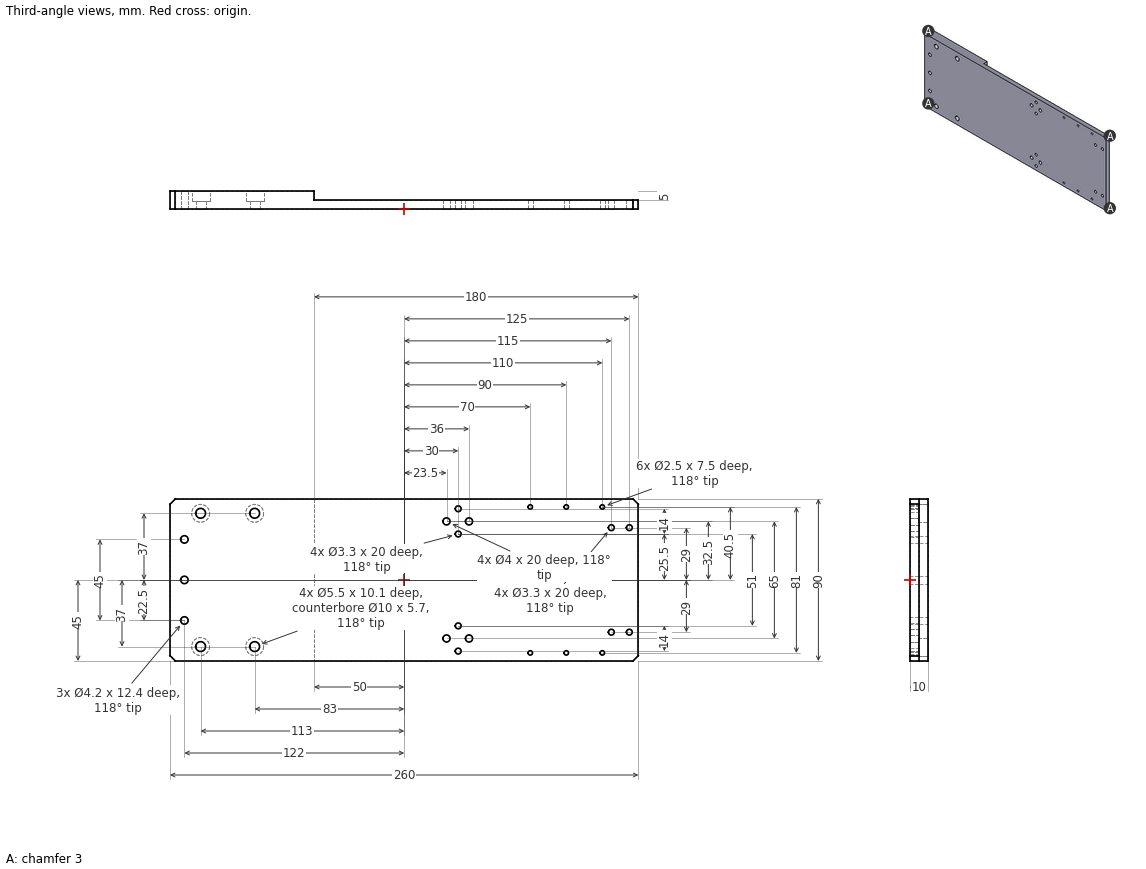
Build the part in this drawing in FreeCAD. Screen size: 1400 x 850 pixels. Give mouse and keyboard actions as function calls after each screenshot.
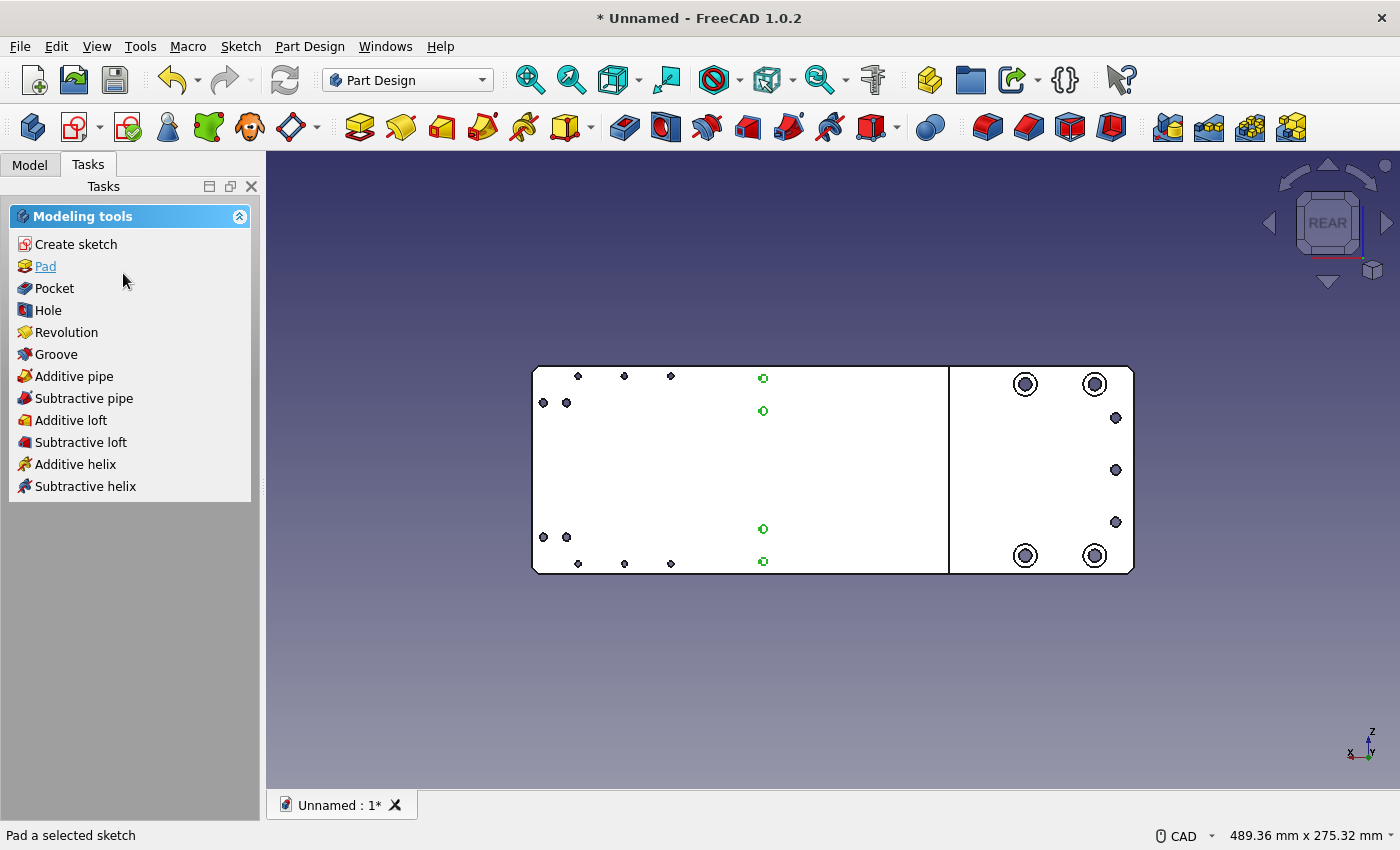
click(666, 128)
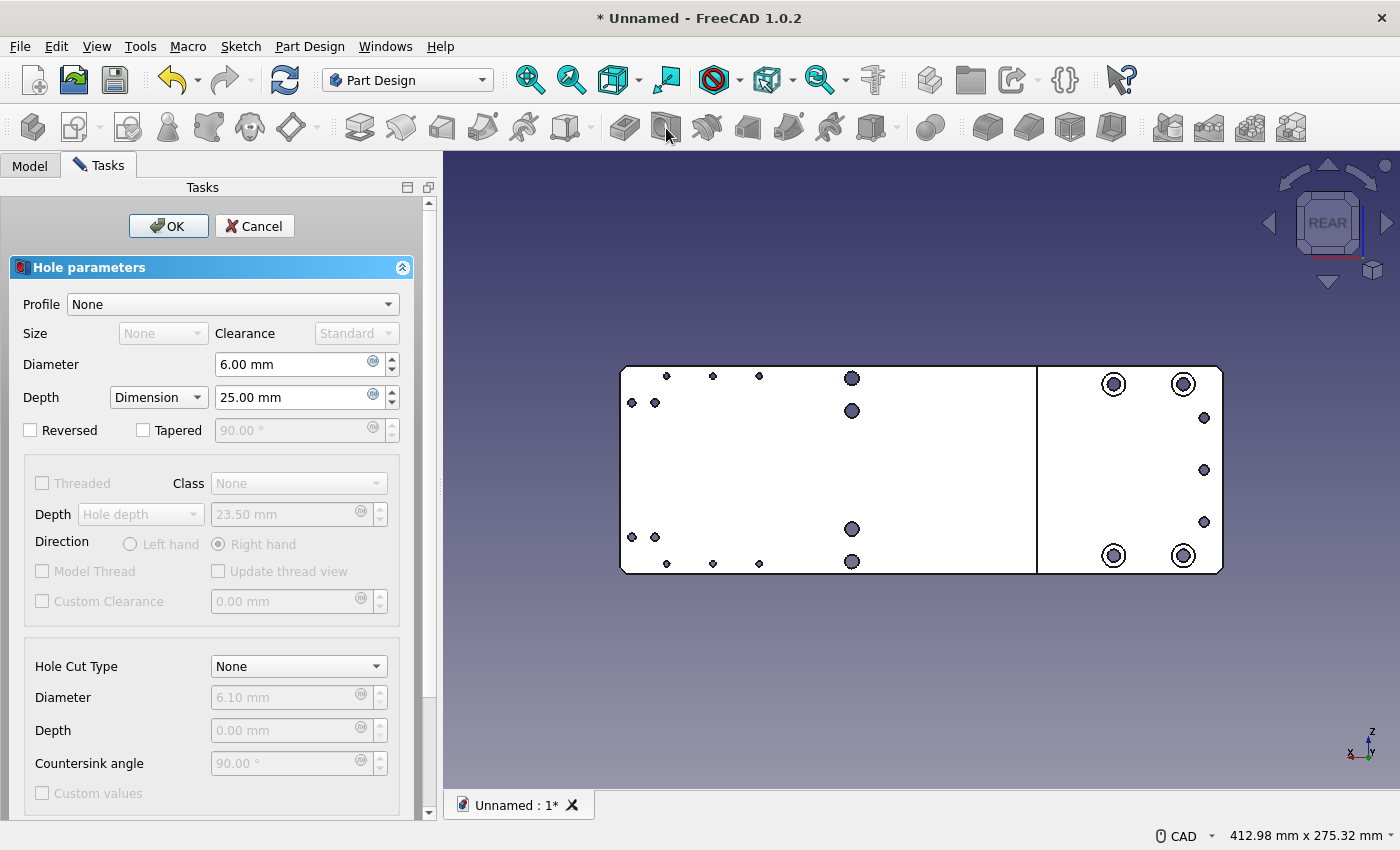
triple_click(300, 364)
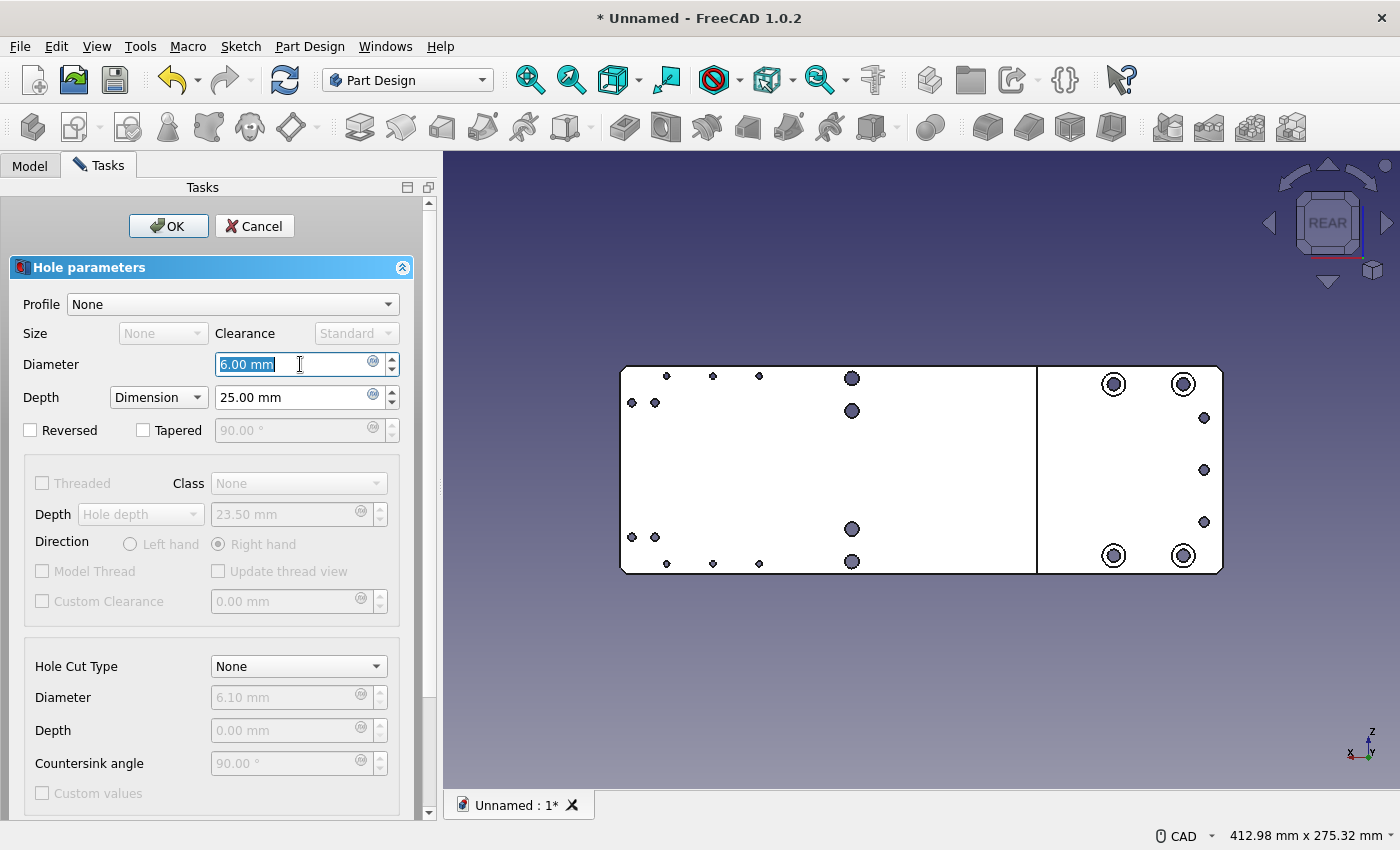
text(3.3)
key(Tab)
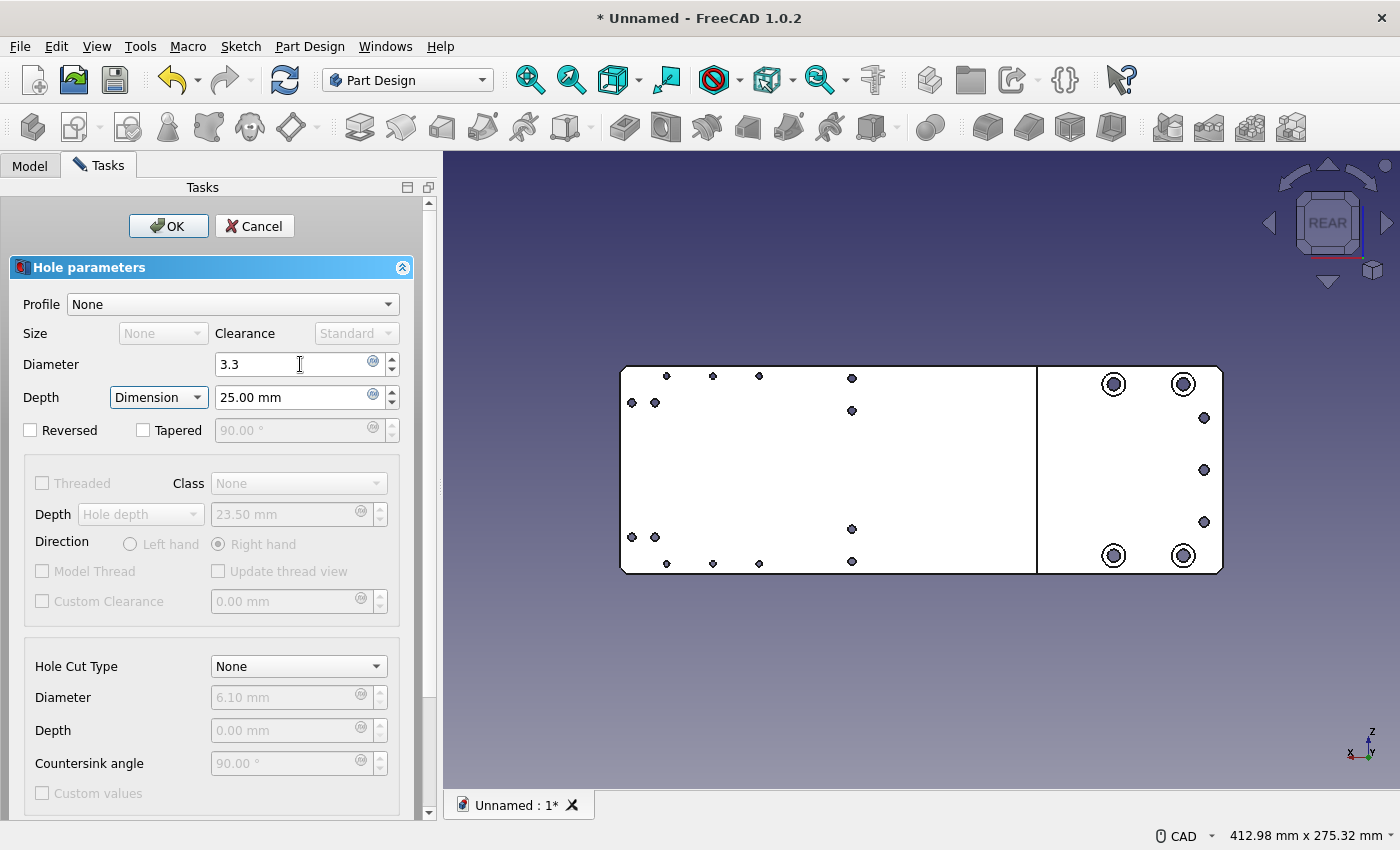
triple_click(300, 398)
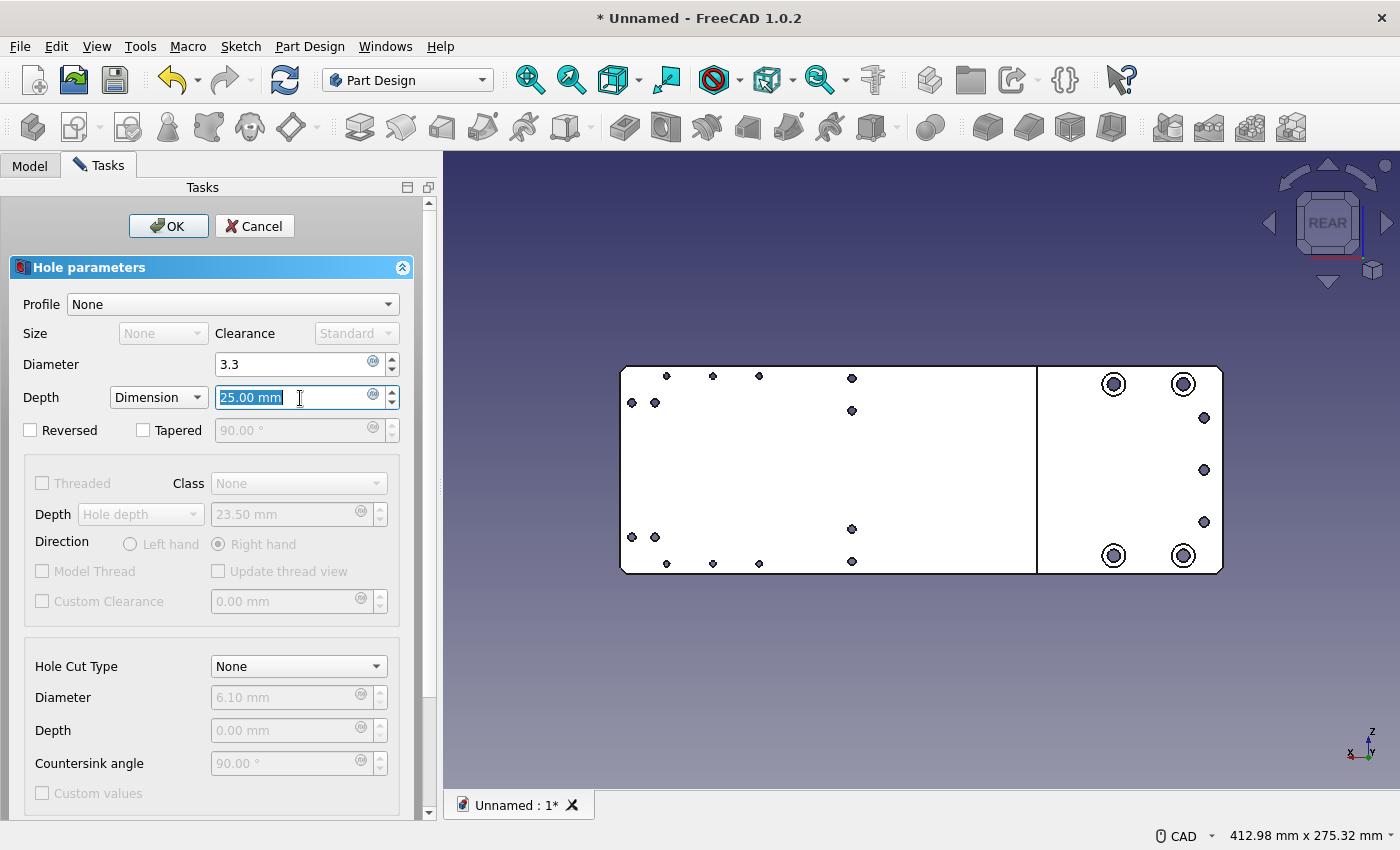
text(20)
key(Tab)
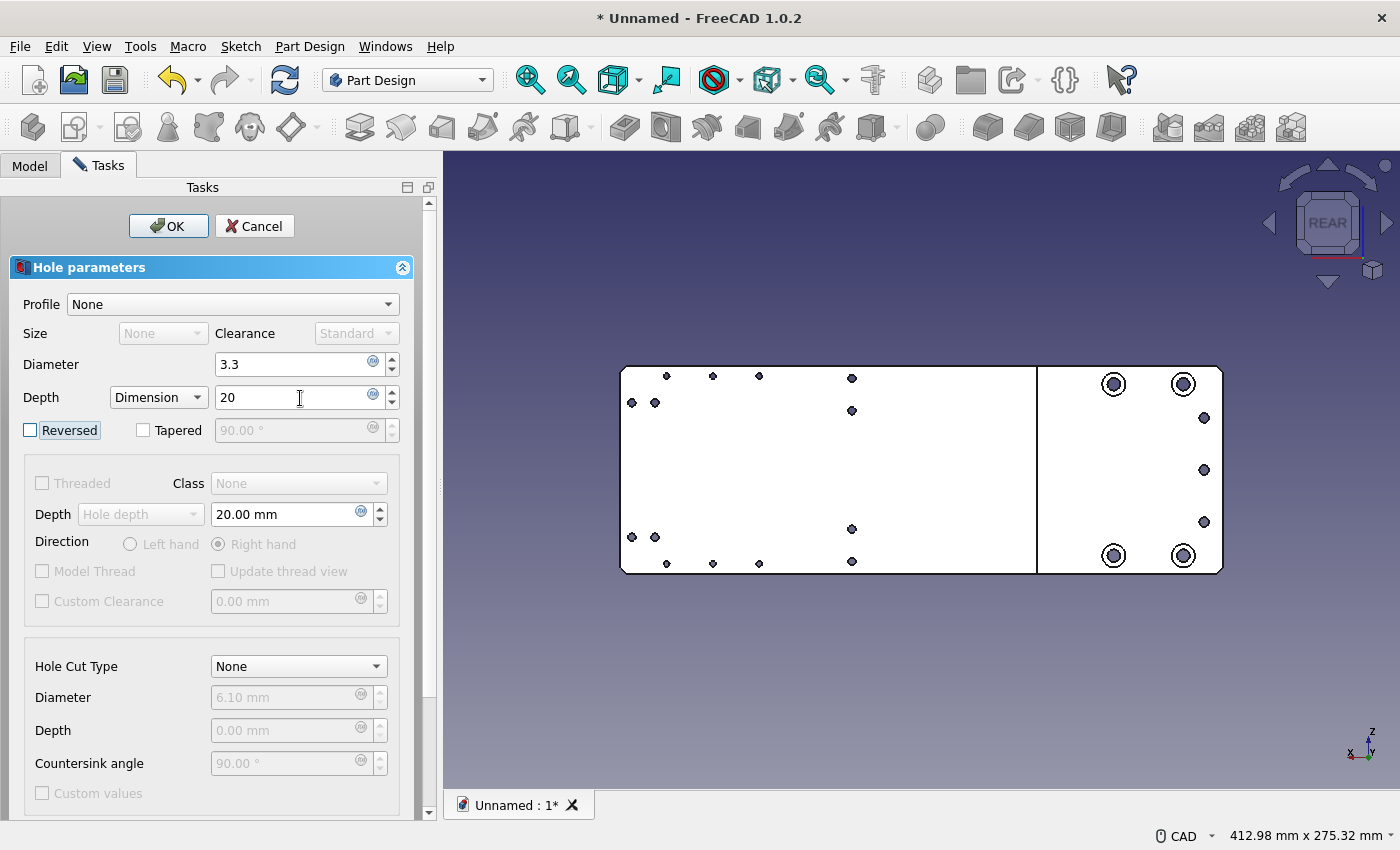
click(169, 226)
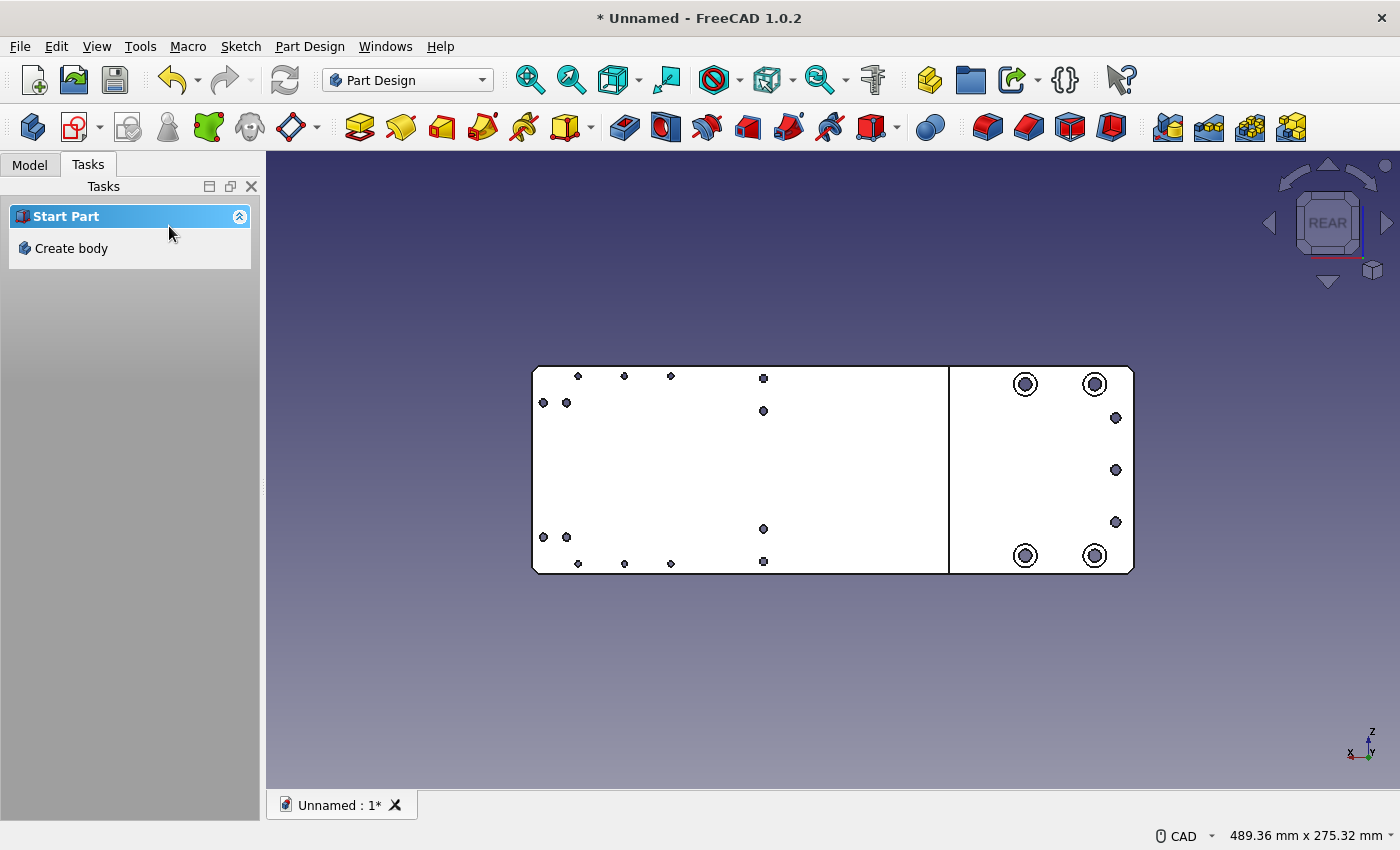
click(681, 469)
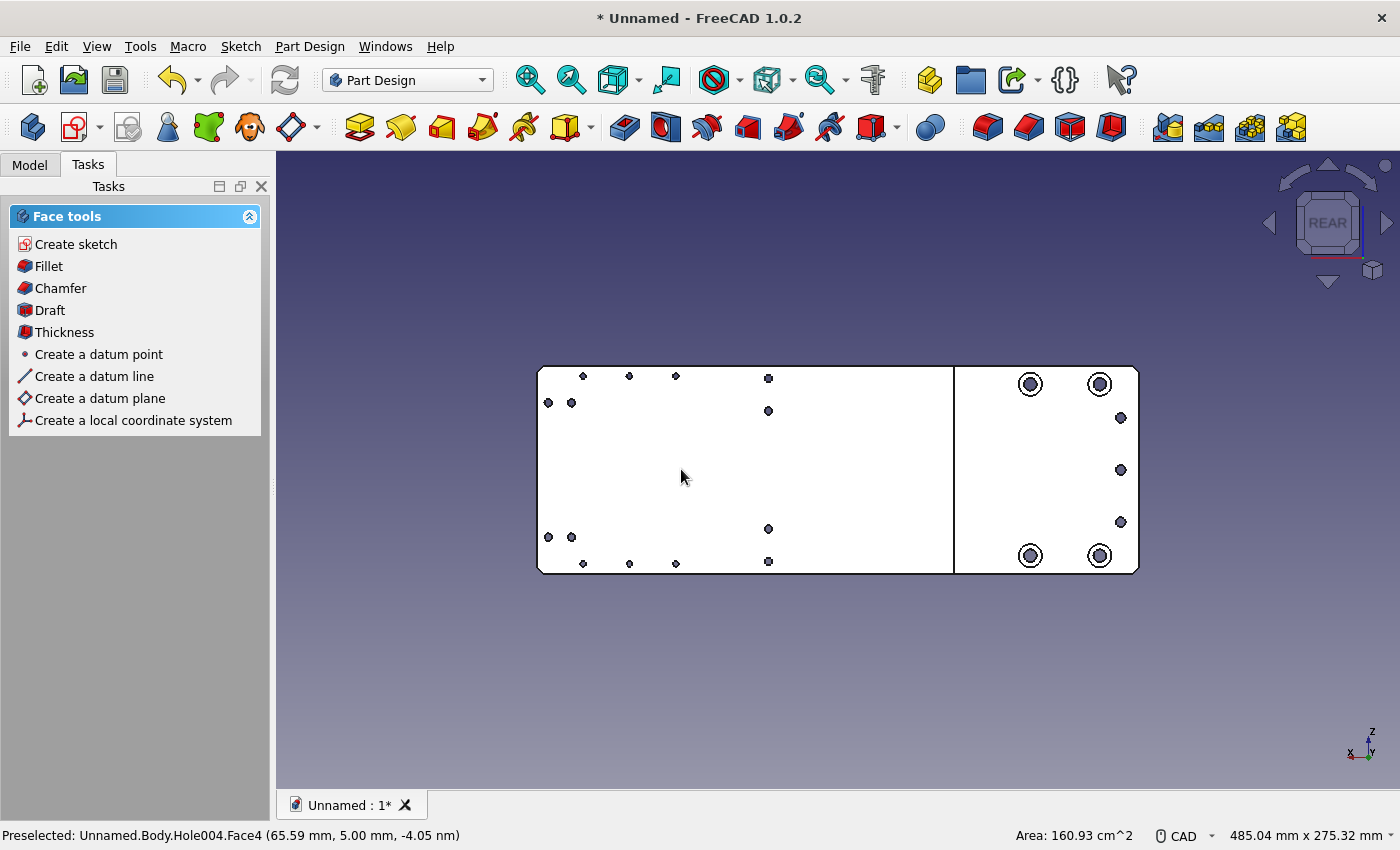
click(74, 128)